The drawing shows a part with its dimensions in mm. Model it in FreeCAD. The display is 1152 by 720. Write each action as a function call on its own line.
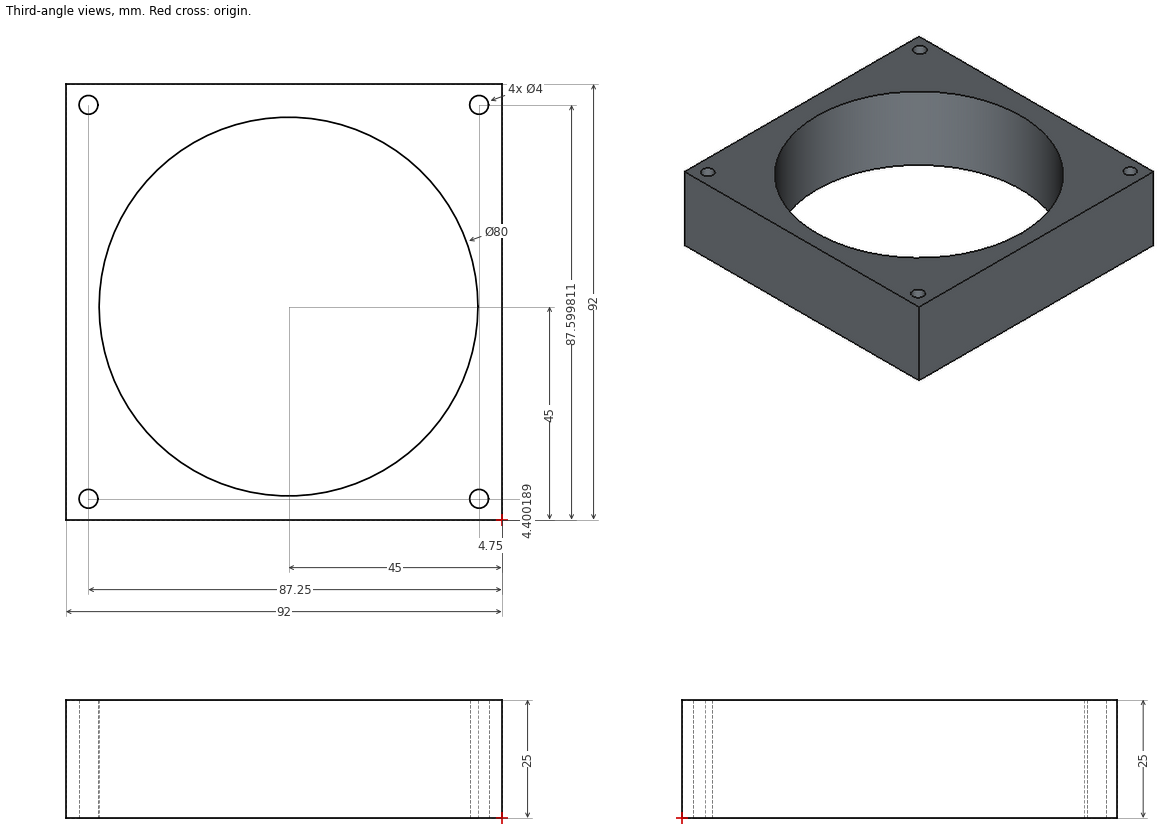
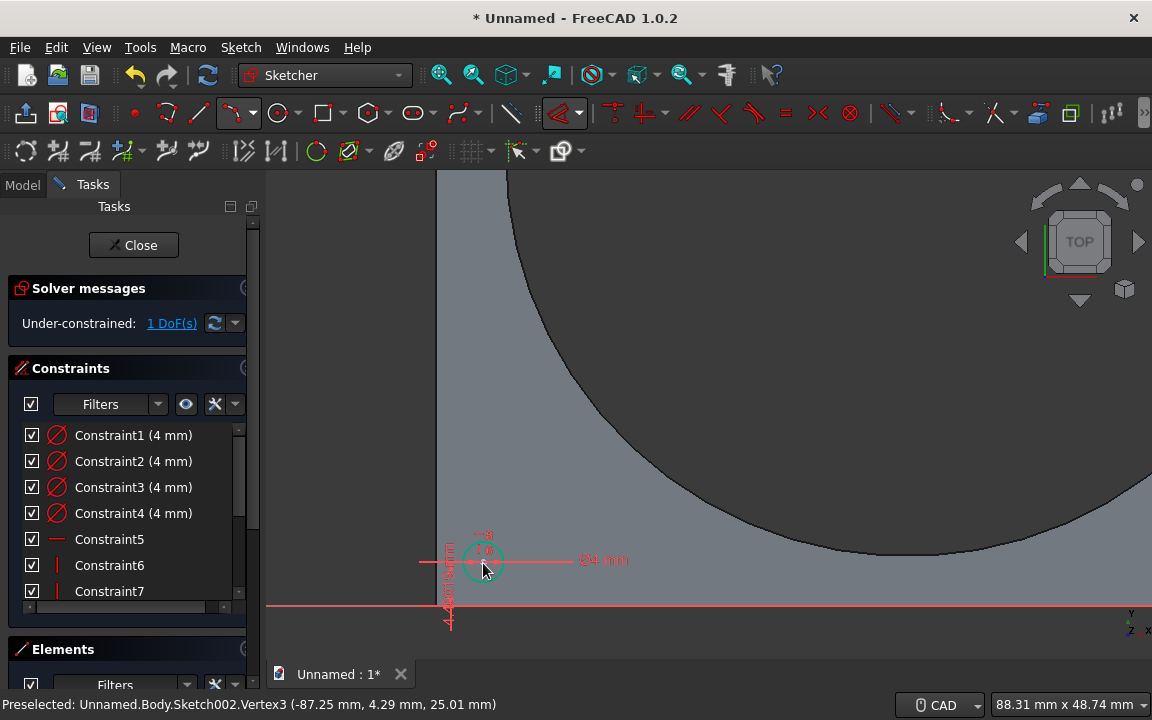
scroll(483, 564, down, 5)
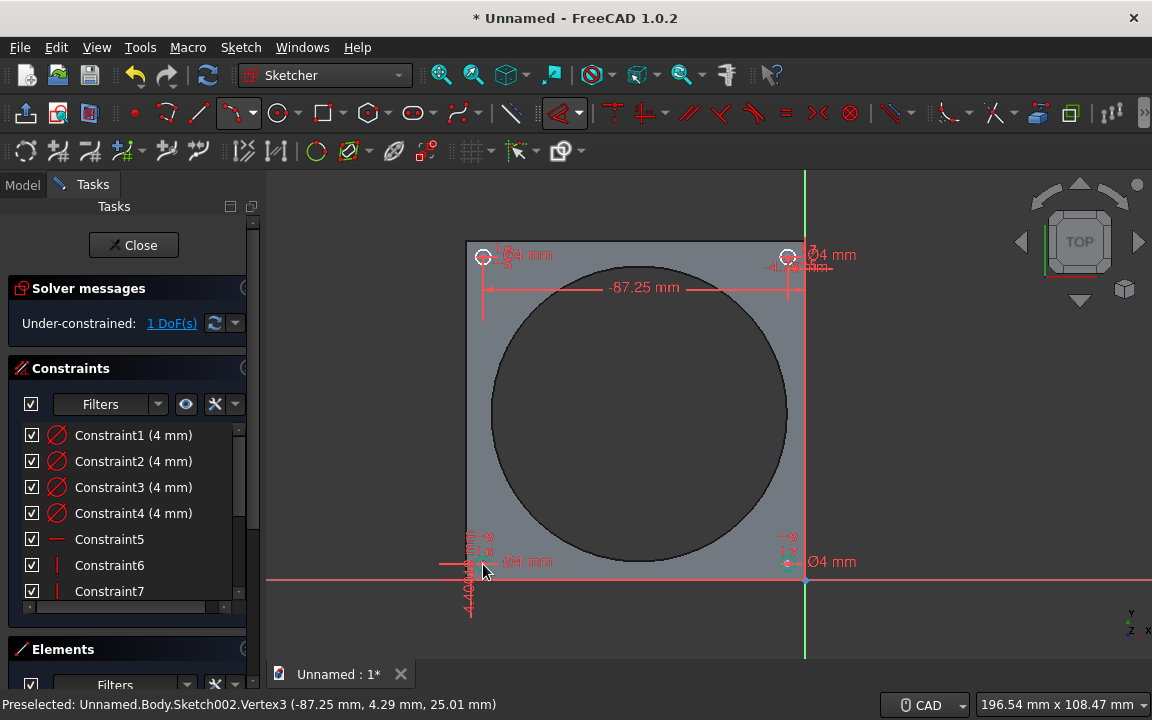
click(788, 257)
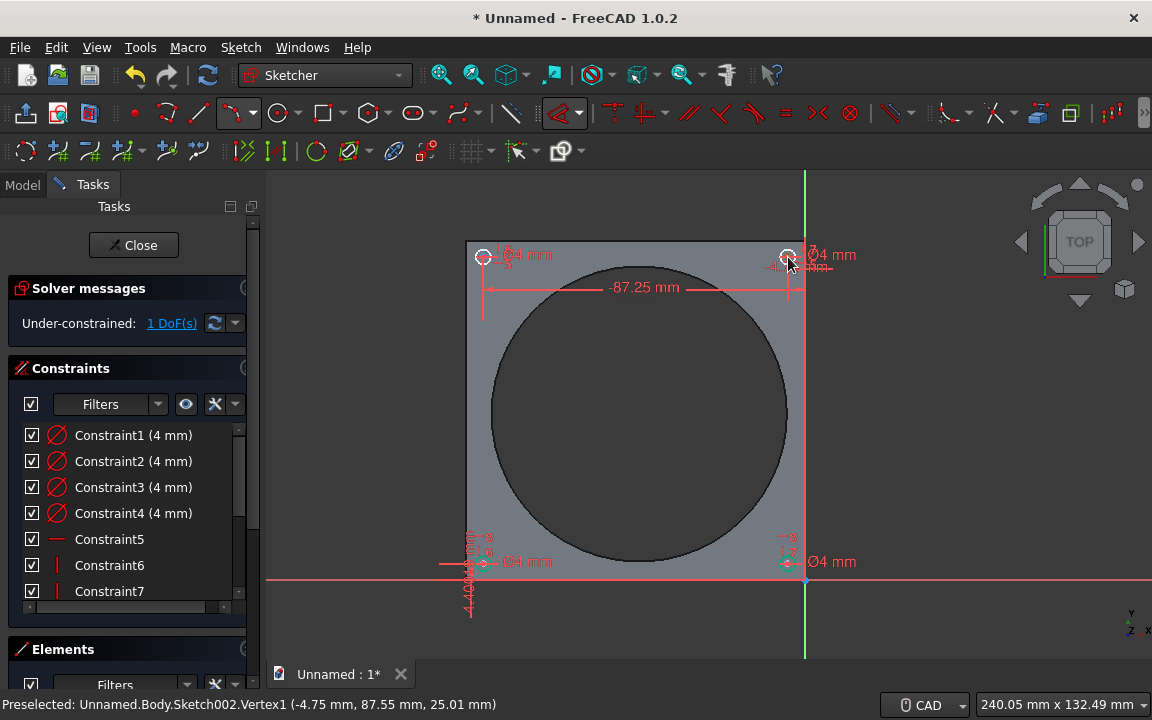
key(i)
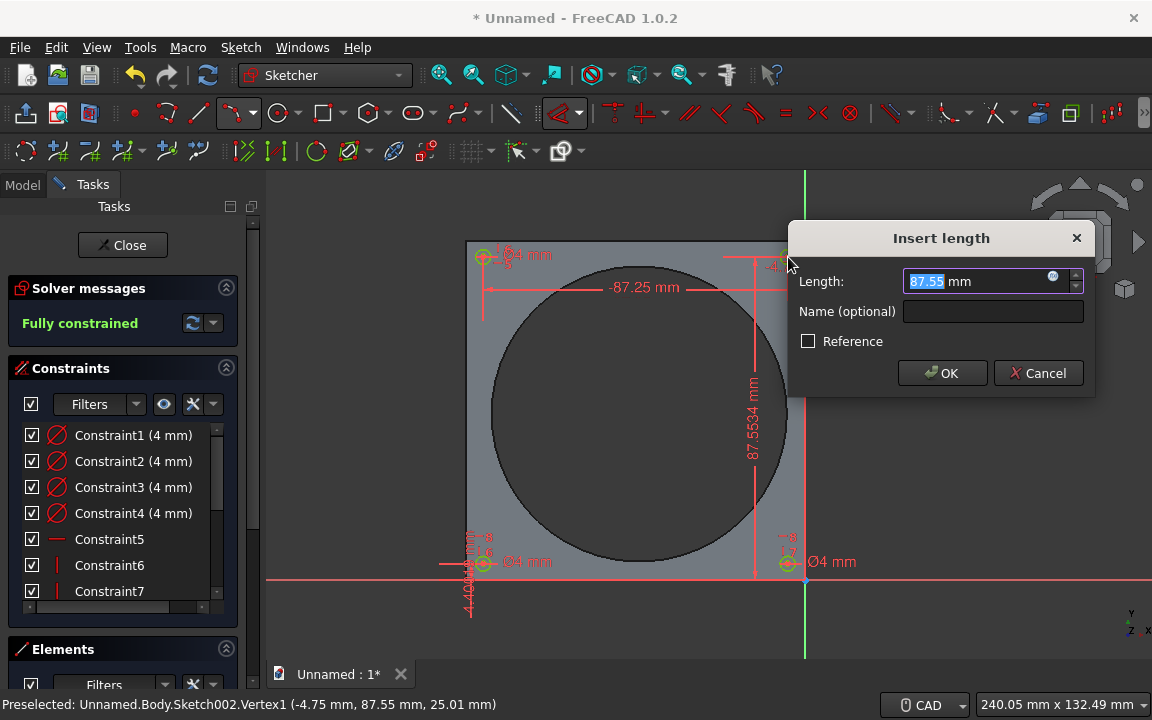
text(87.599811)
key(Return)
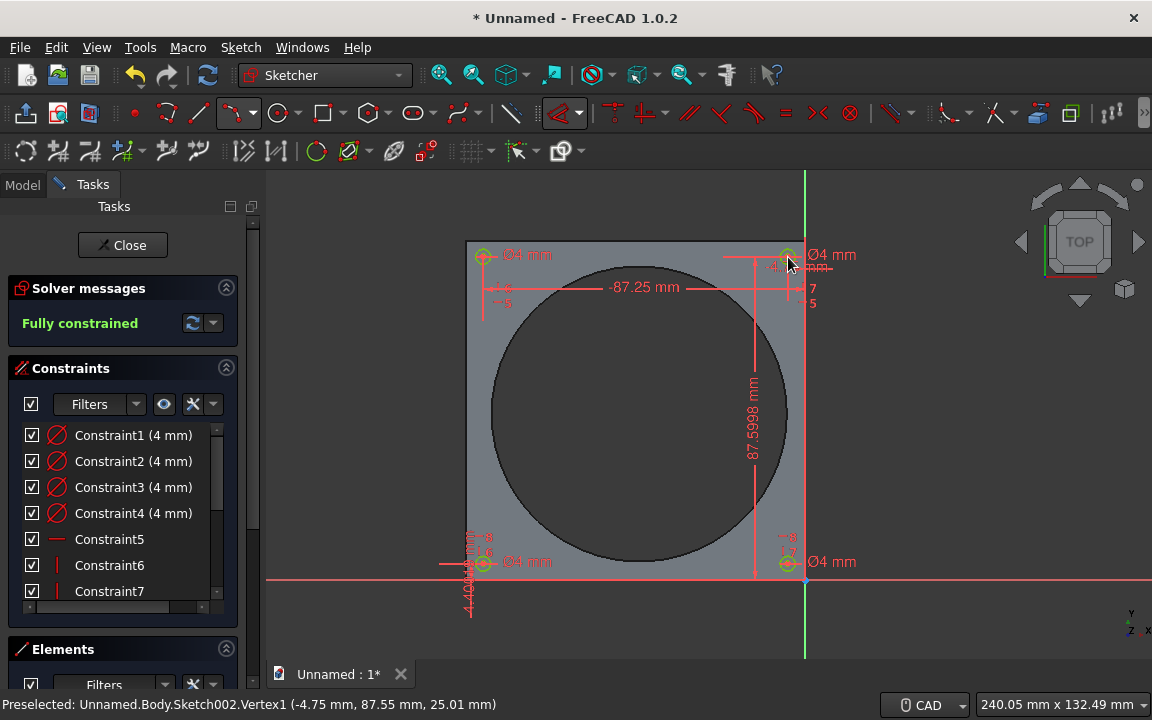
click(123, 245)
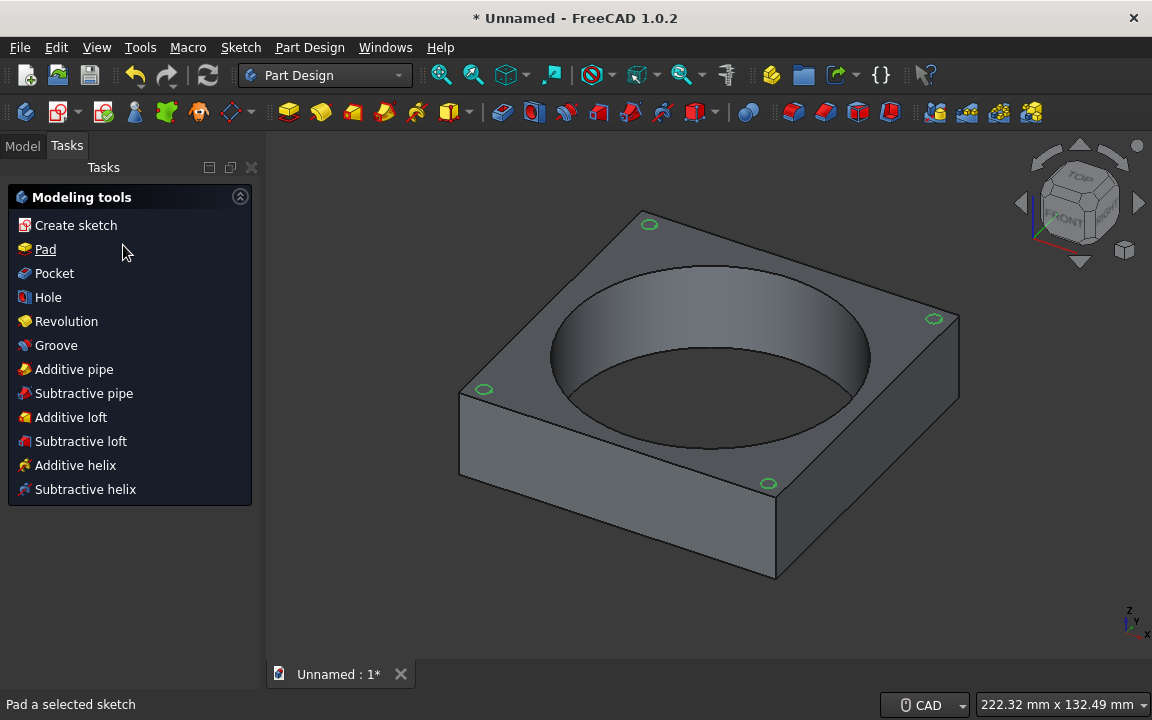
click(504, 112)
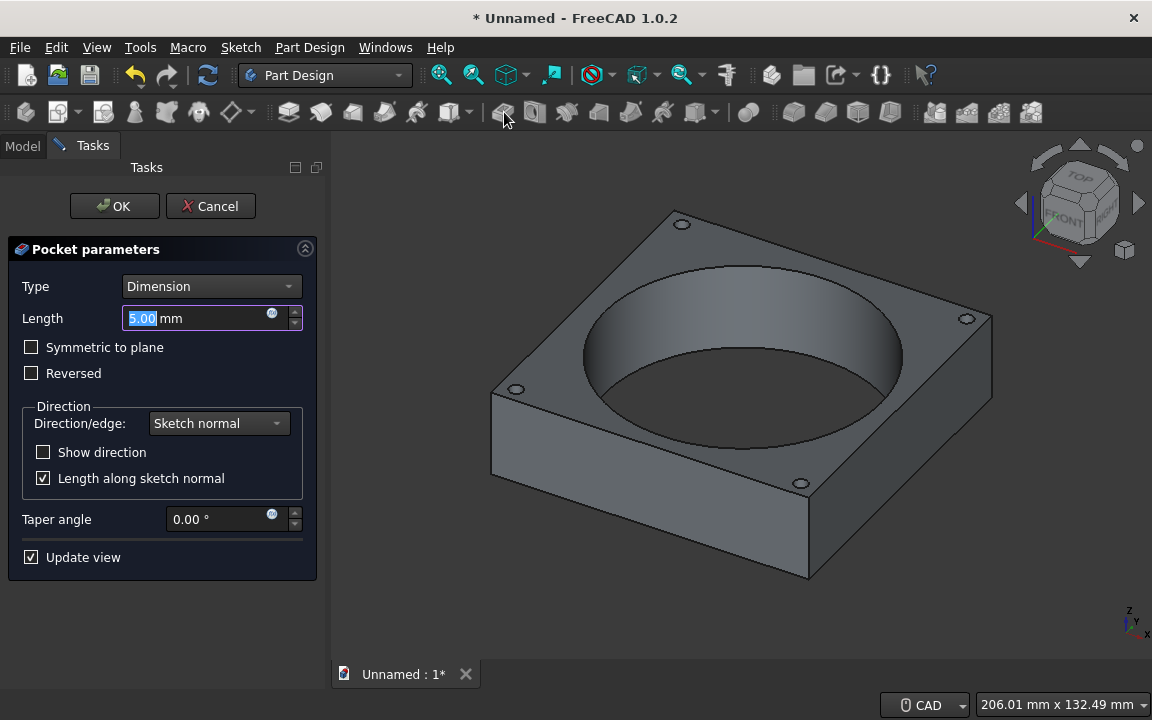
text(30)
key(Tab)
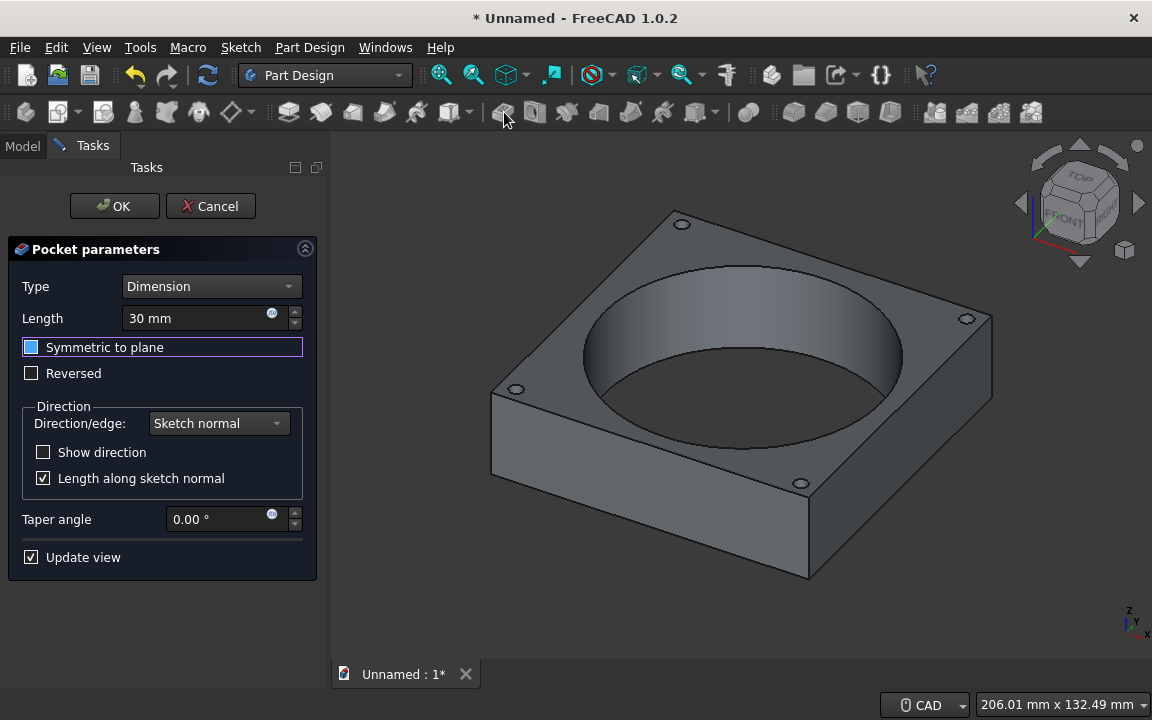
click(115, 206)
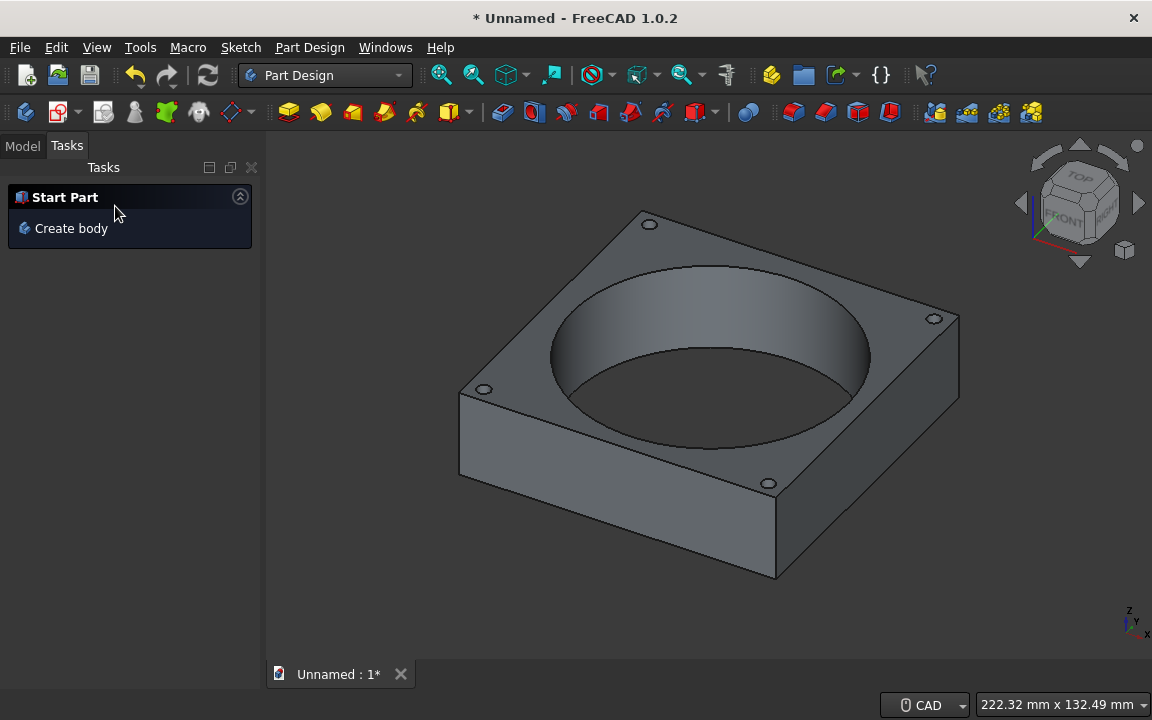
key(0)